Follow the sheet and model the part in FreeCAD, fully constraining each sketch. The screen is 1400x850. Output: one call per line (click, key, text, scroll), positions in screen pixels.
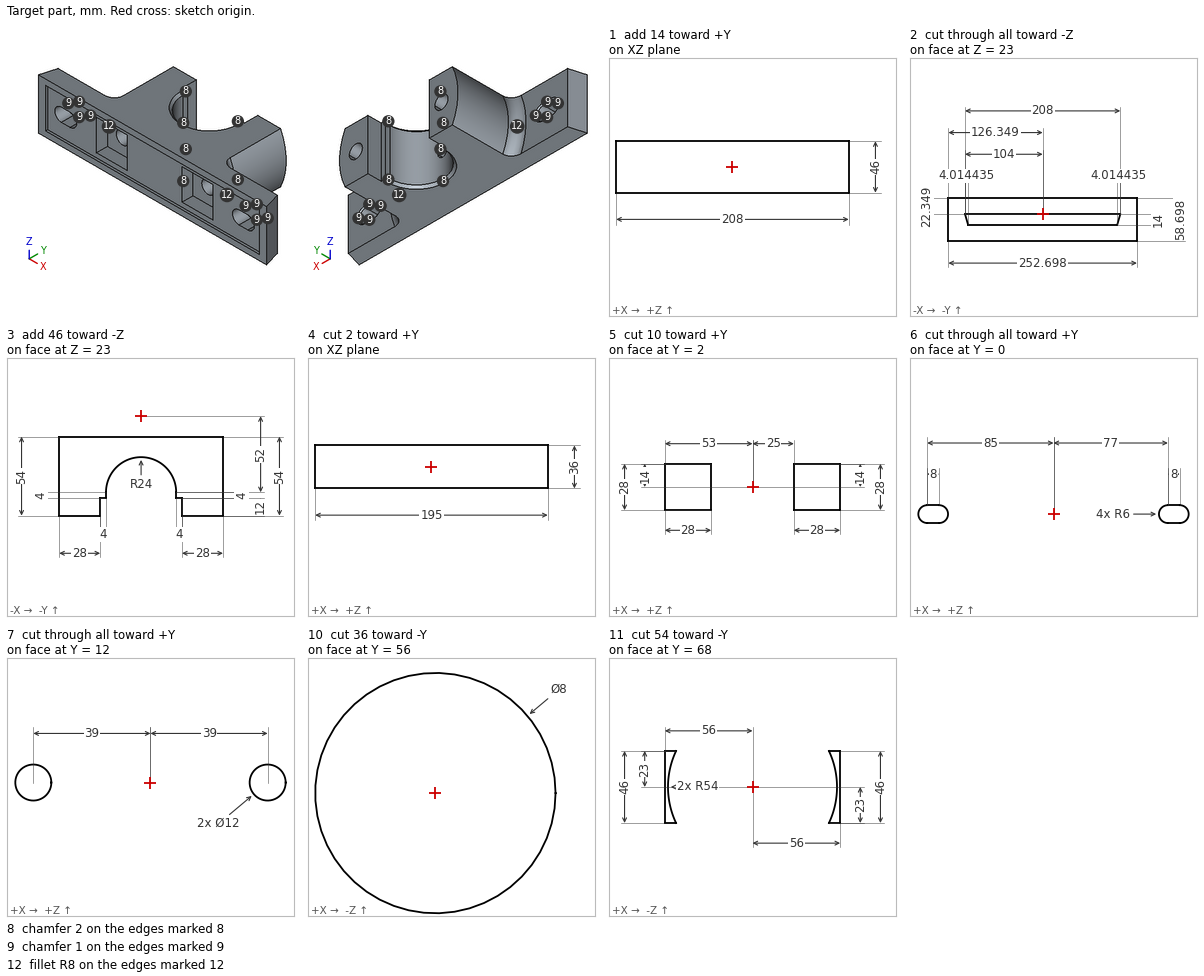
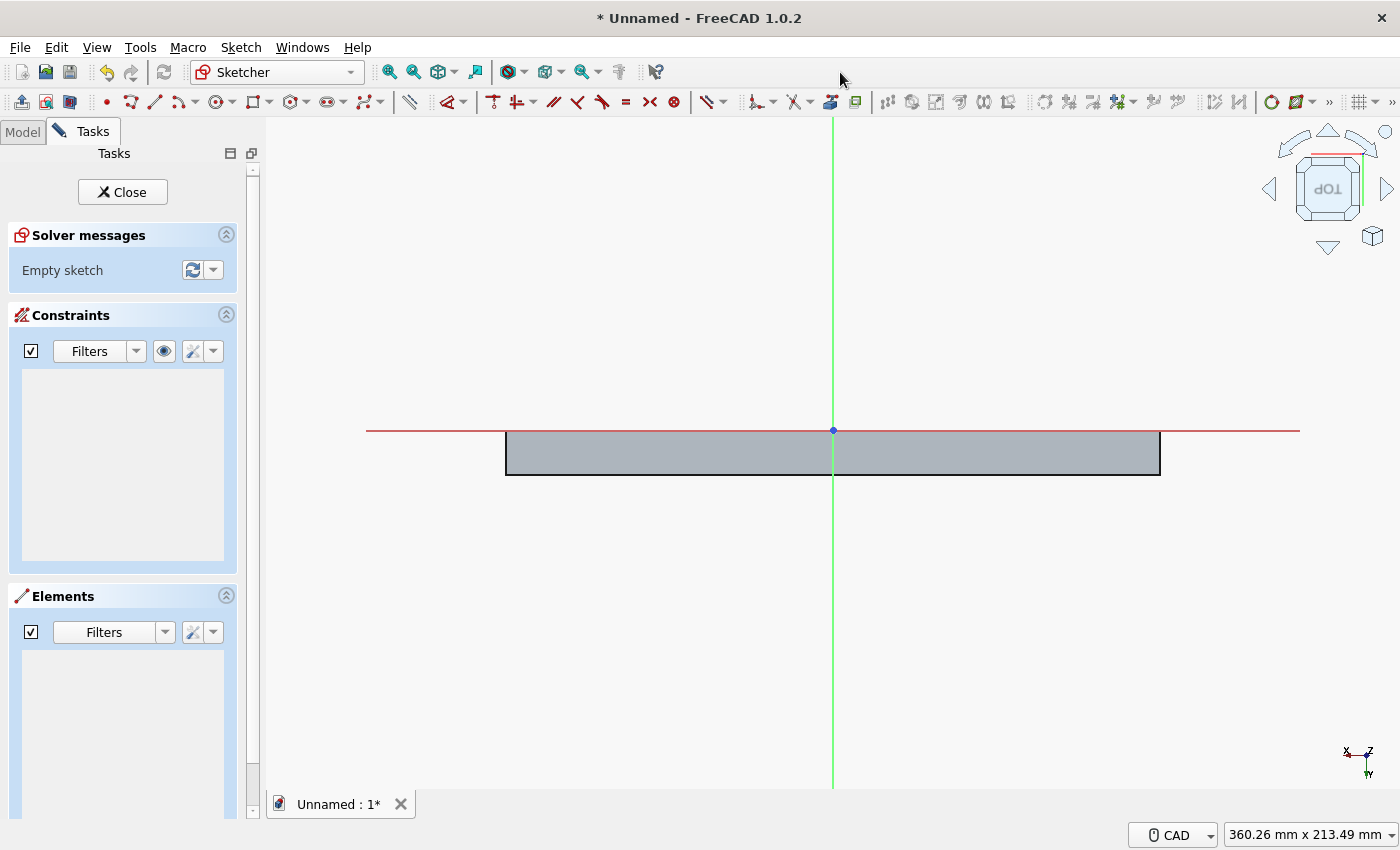
scroll(455, 453, down, 1)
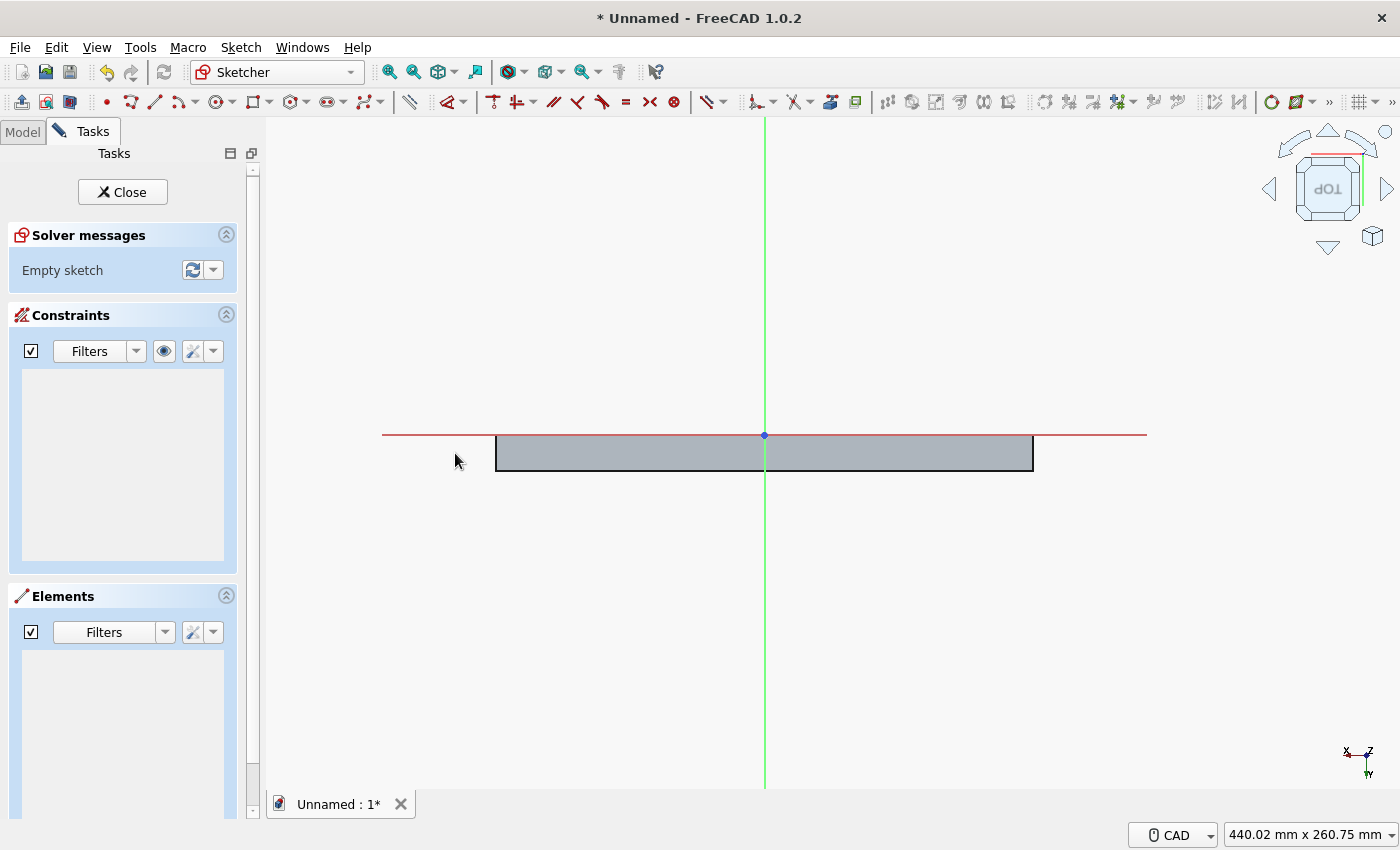
click(254, 102)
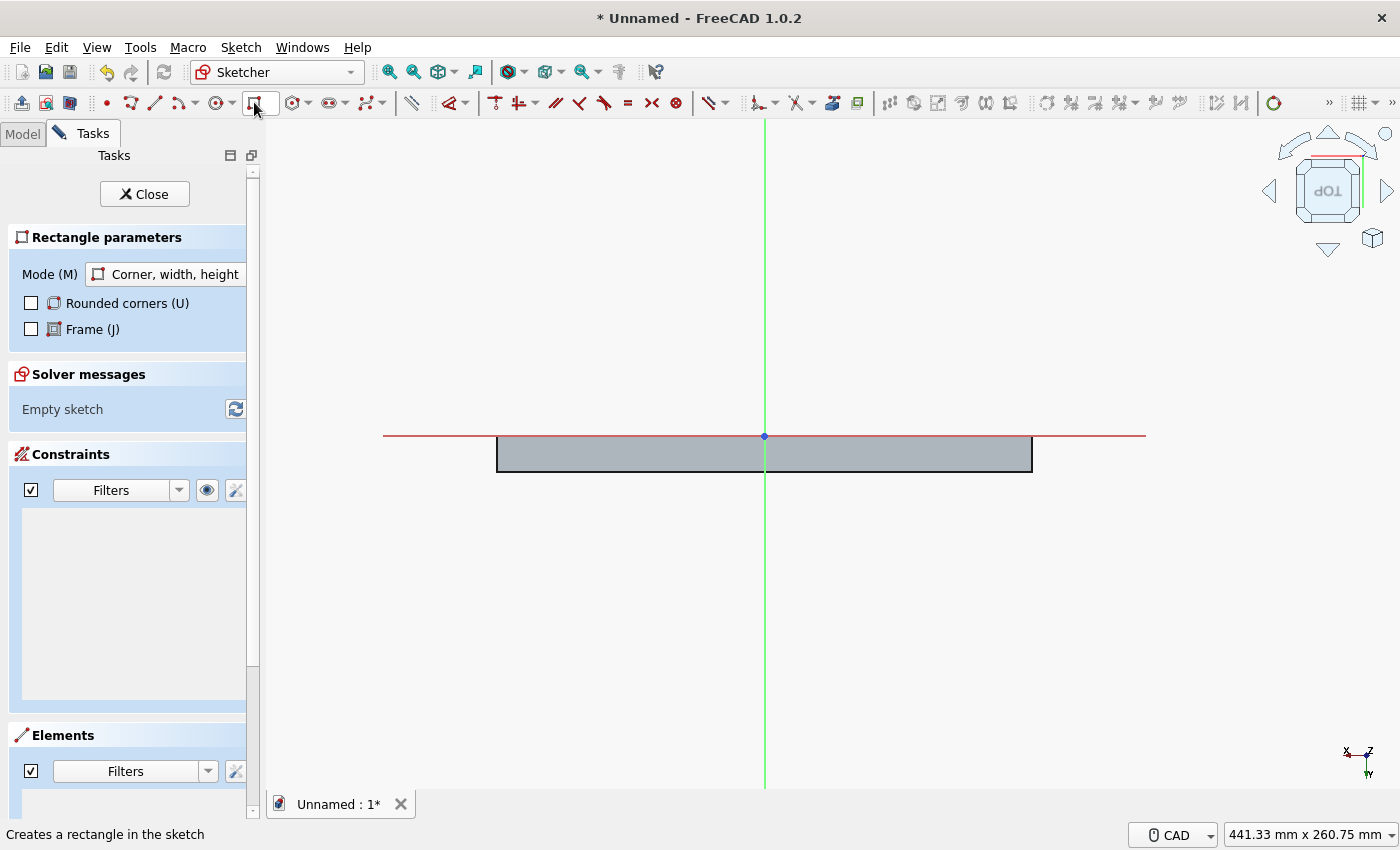
click(440, 379)
move(1089, 530)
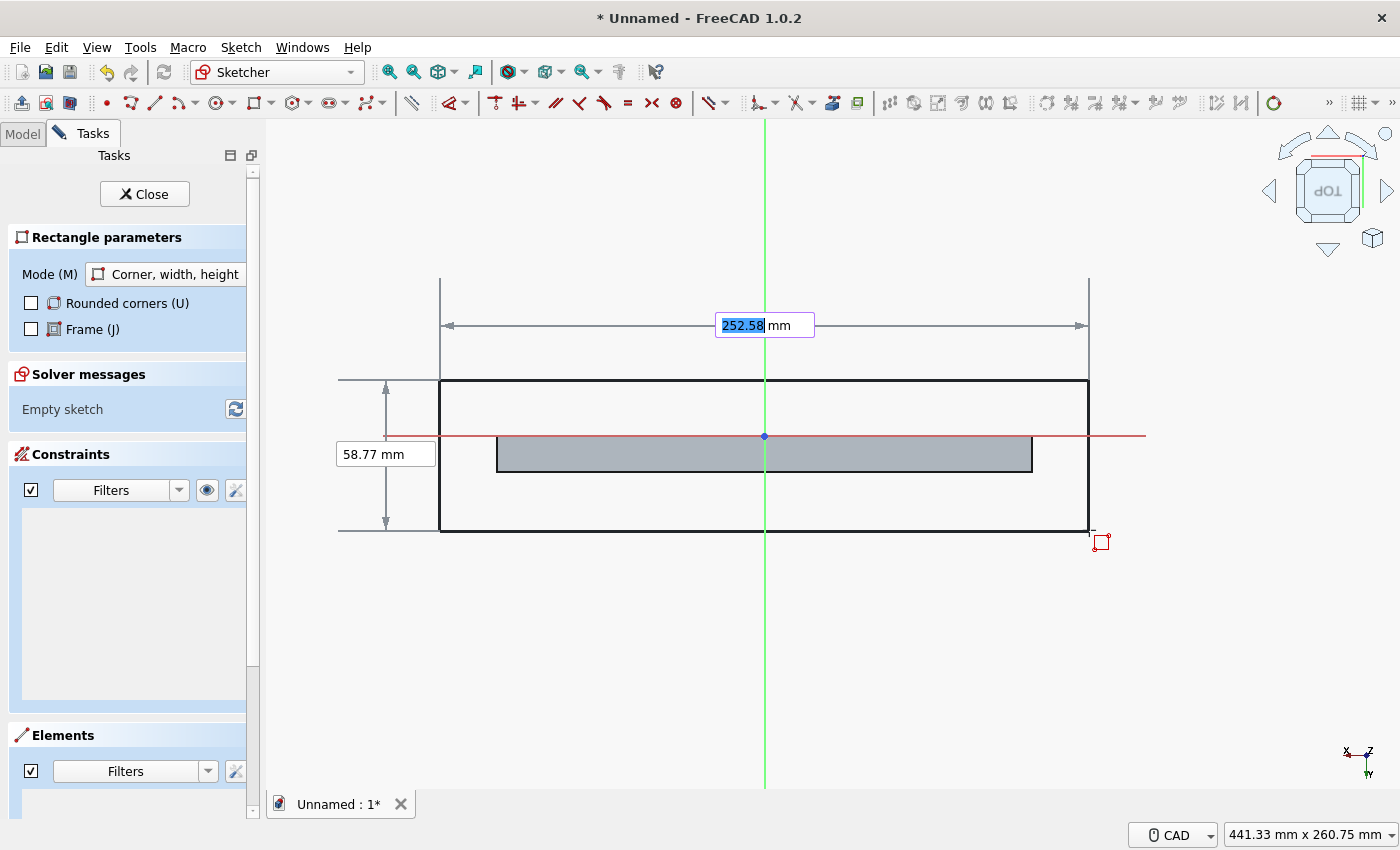
text(252.698)
key(Tab)
text(58.698)
key(Return)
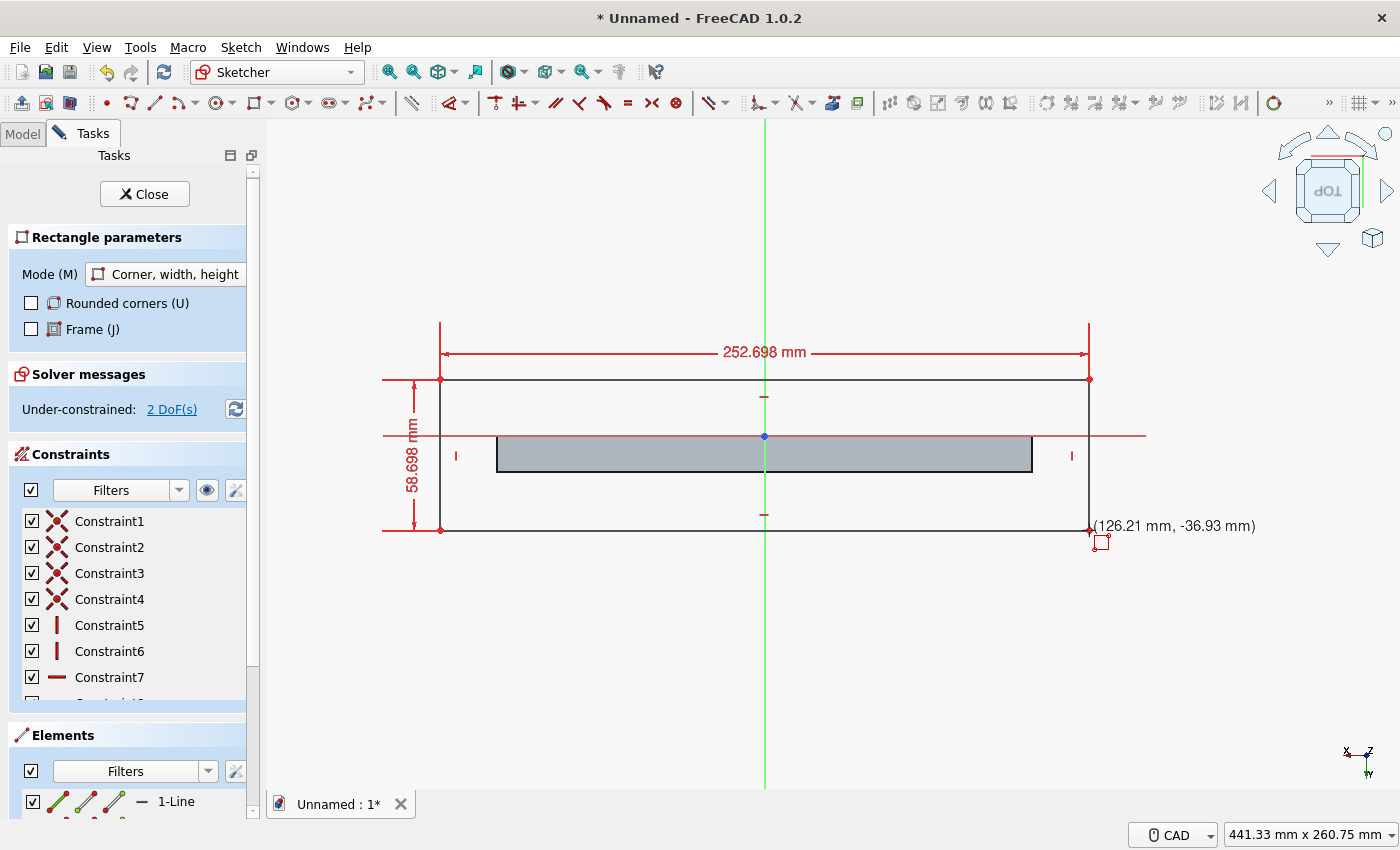
key(g)
key(m)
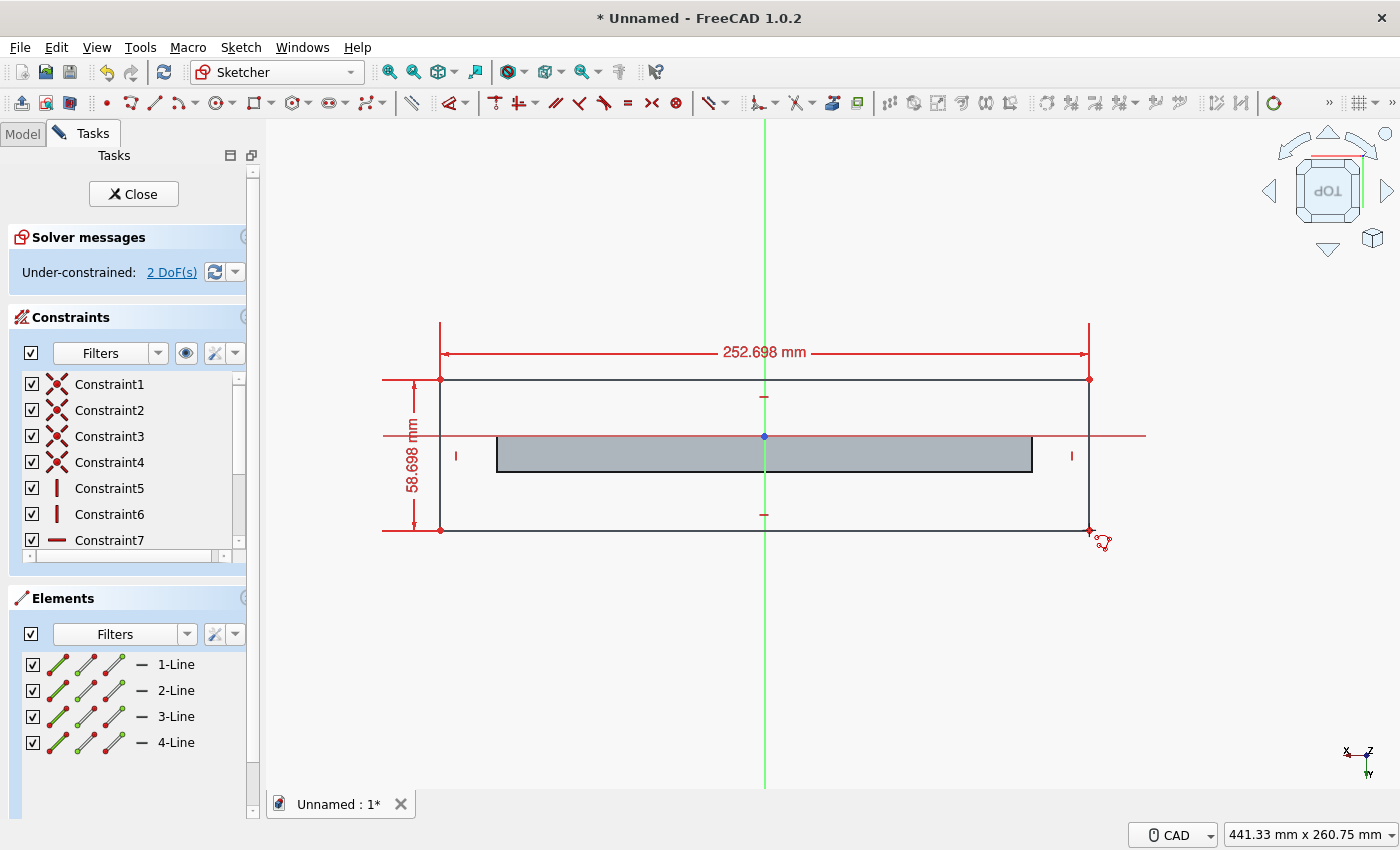
click(1022, 472)
click(508, 472)
click(497, 436)
click(1032, 445)
click(1022, 473)
key(Escape)
key(Escape)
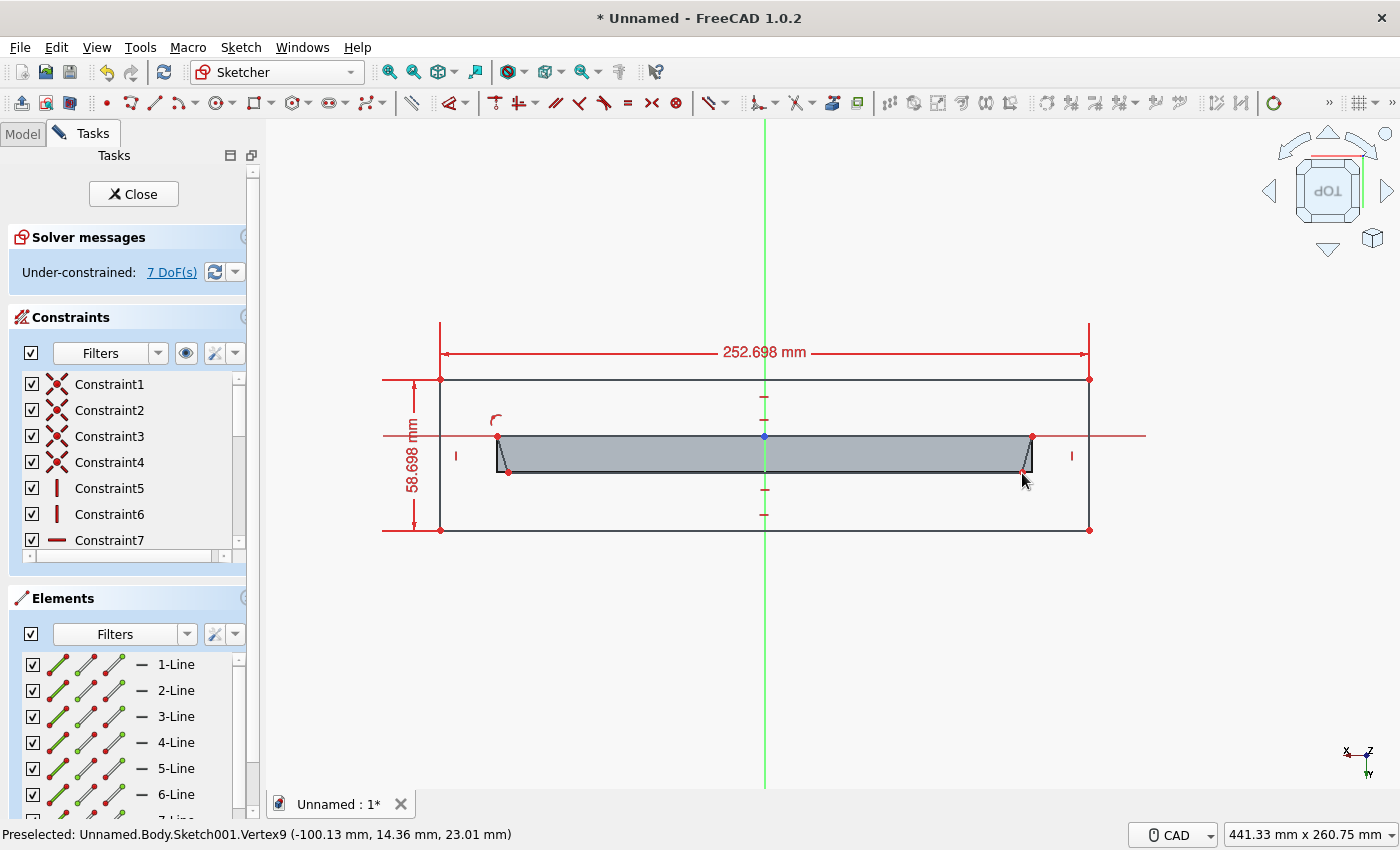
key(d)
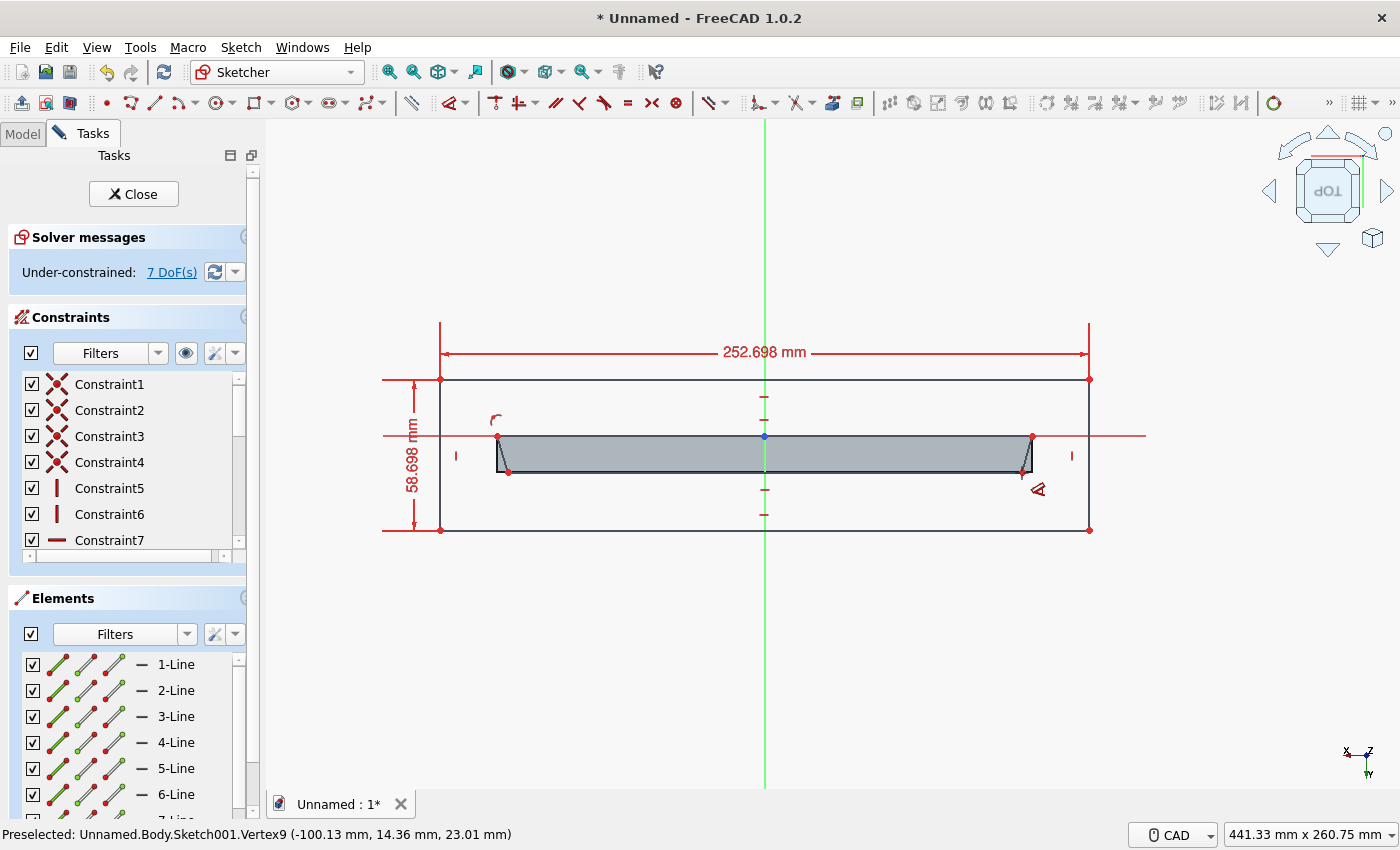
click(657, 436)
click(641, 402)